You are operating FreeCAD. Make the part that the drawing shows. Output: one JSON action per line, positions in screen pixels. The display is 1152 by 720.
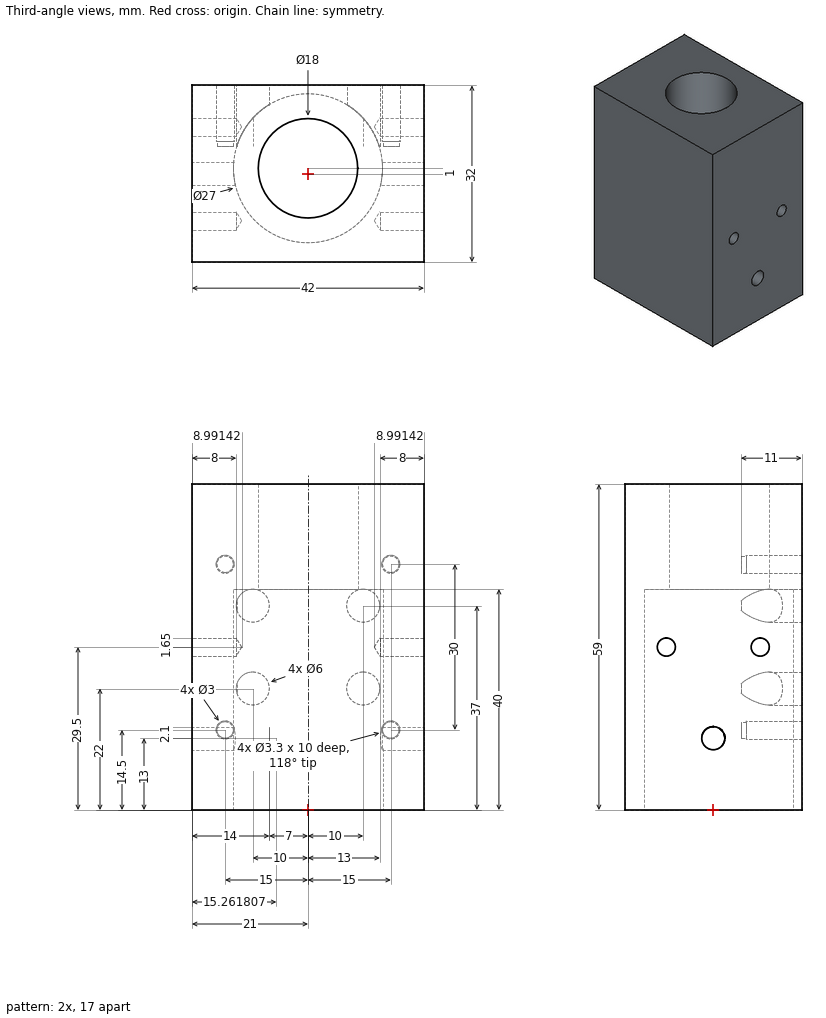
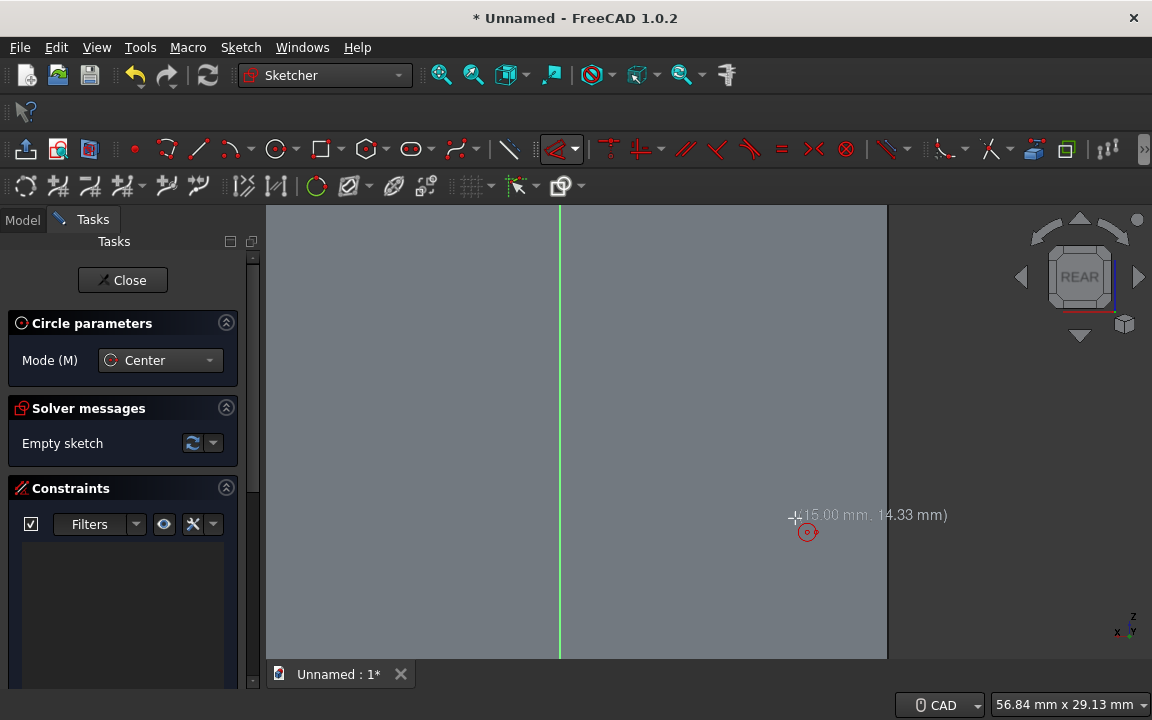
{"action": "left_click", "coordinate": [794, 517]}
{"action": "left_click", "coordinate": [811, 500]}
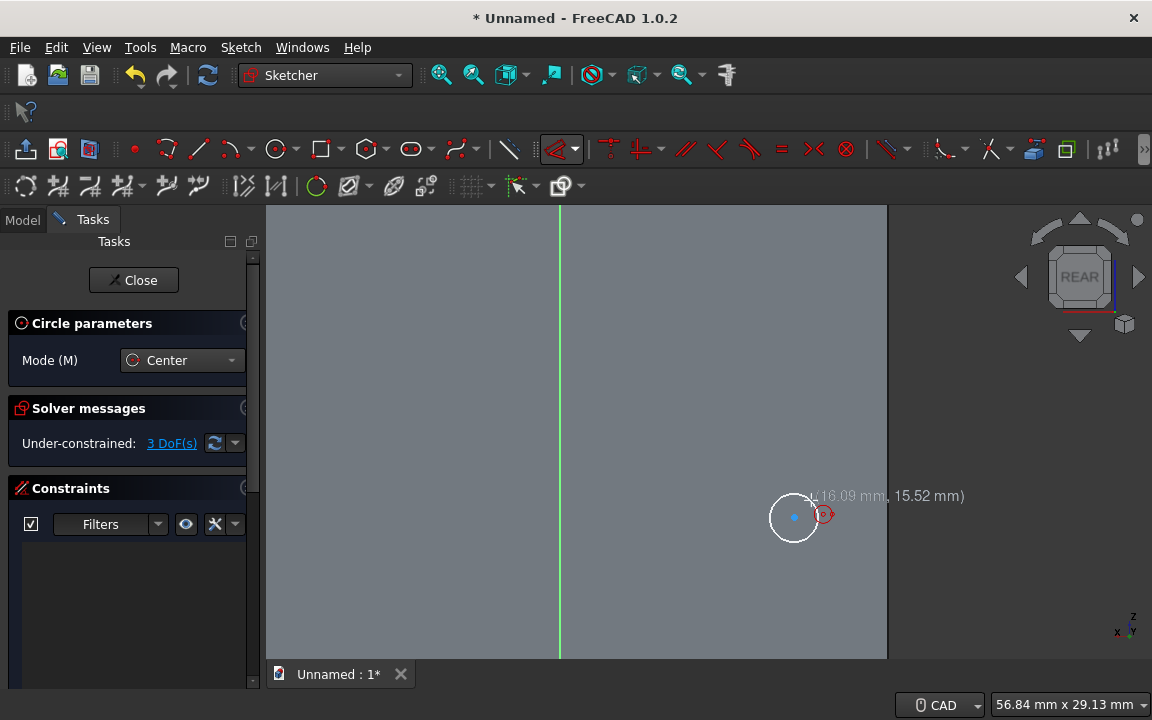
{"action": "left_click", "coordinate": [716, 400]}
{"action": "left_click", "coordinate": [749, 367]}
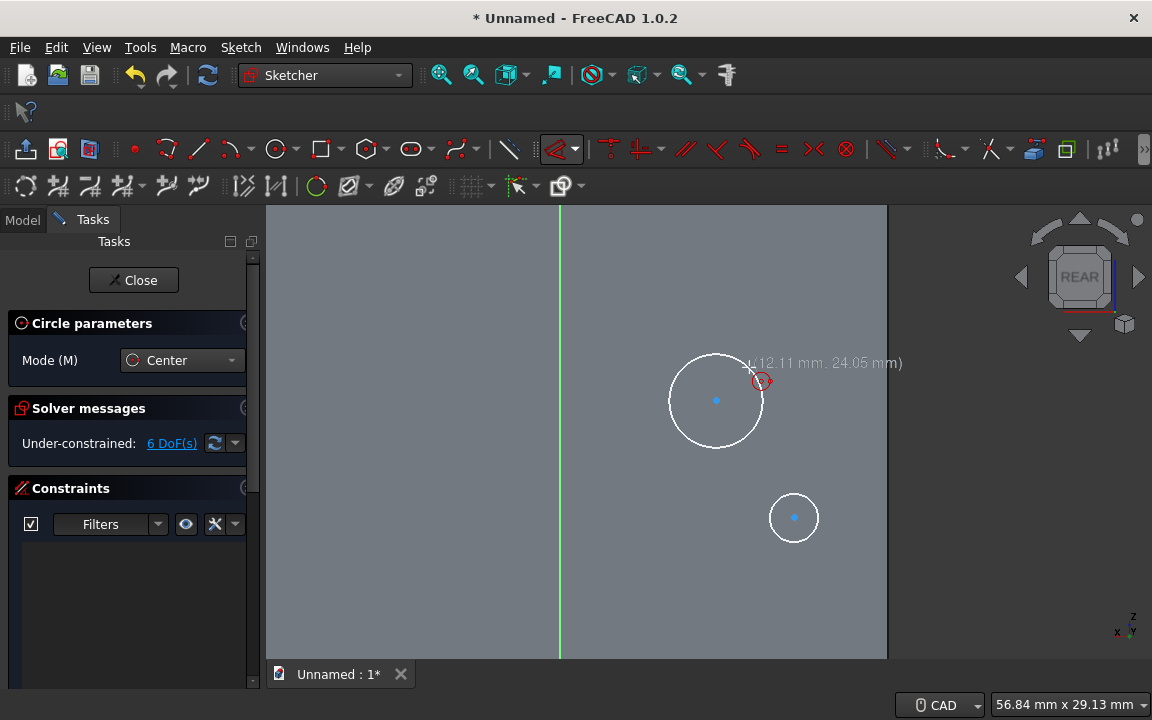
{"action": "left_click", "coordinate": [404, 400]}
{"action": "left_click", "coordinate": [437, 367]}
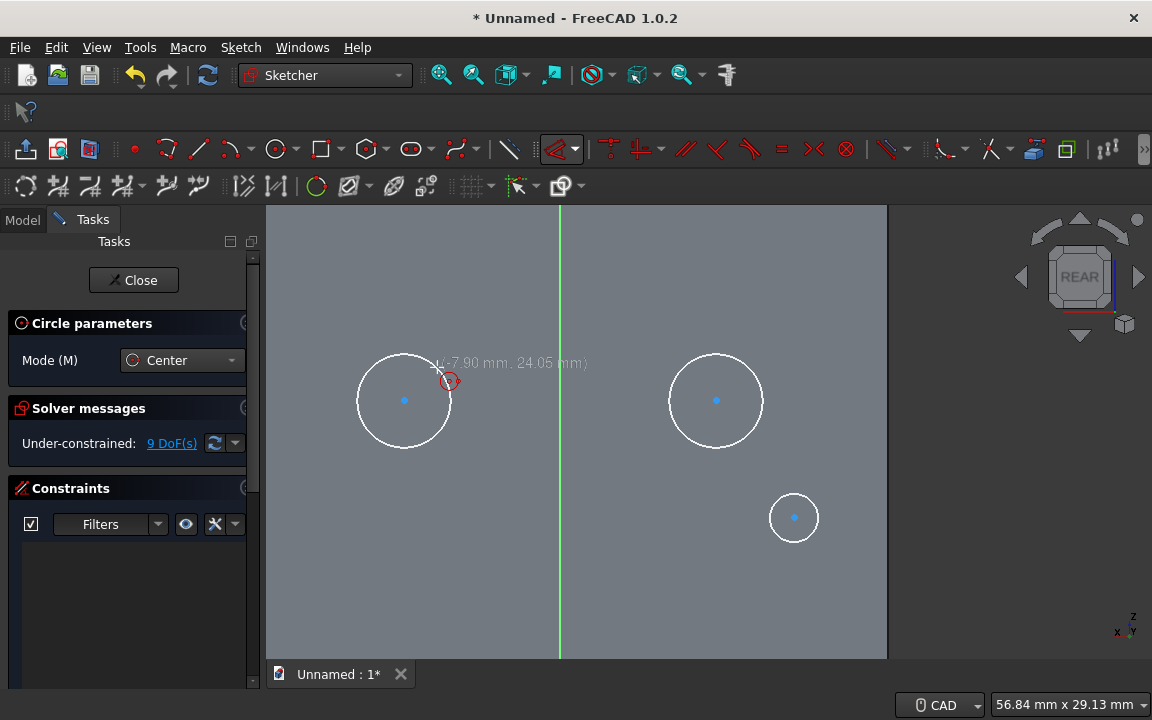
{"action": "left_click", "coordinate": [326, 517]}
{"action": "left_click", "coordinate": [343, 500]}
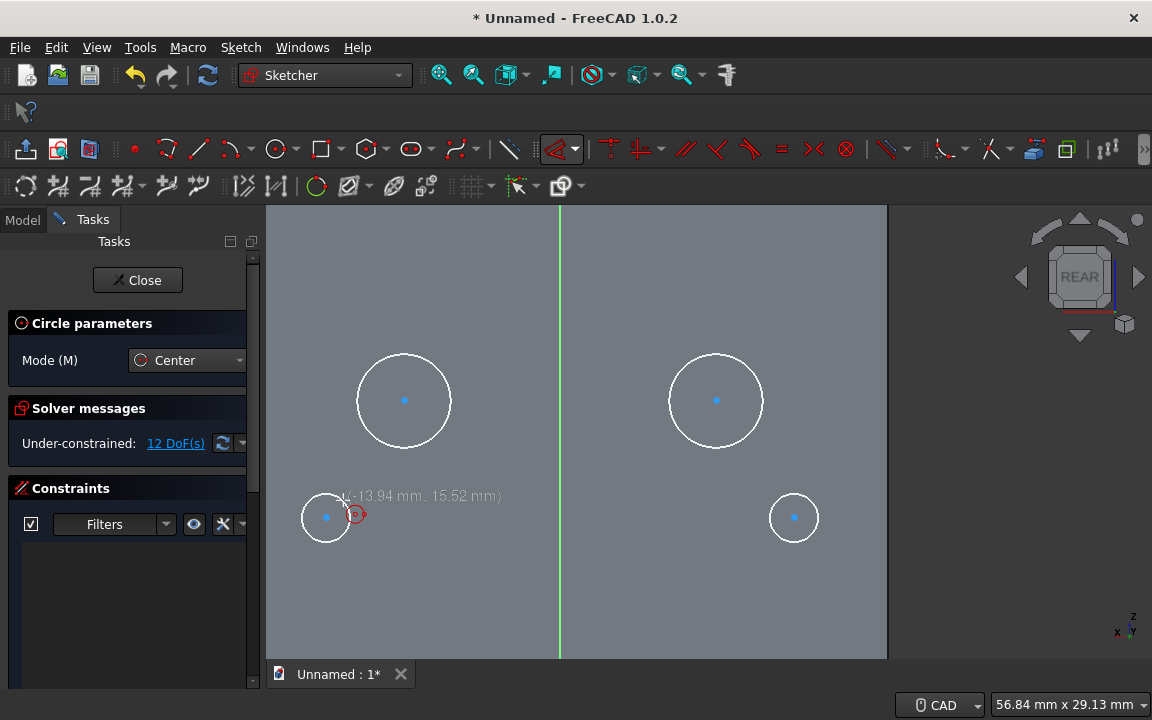
{"action": "scroll", "coordinate": [687, 460], "scroll_direction": "down", "scroll_amount": 5}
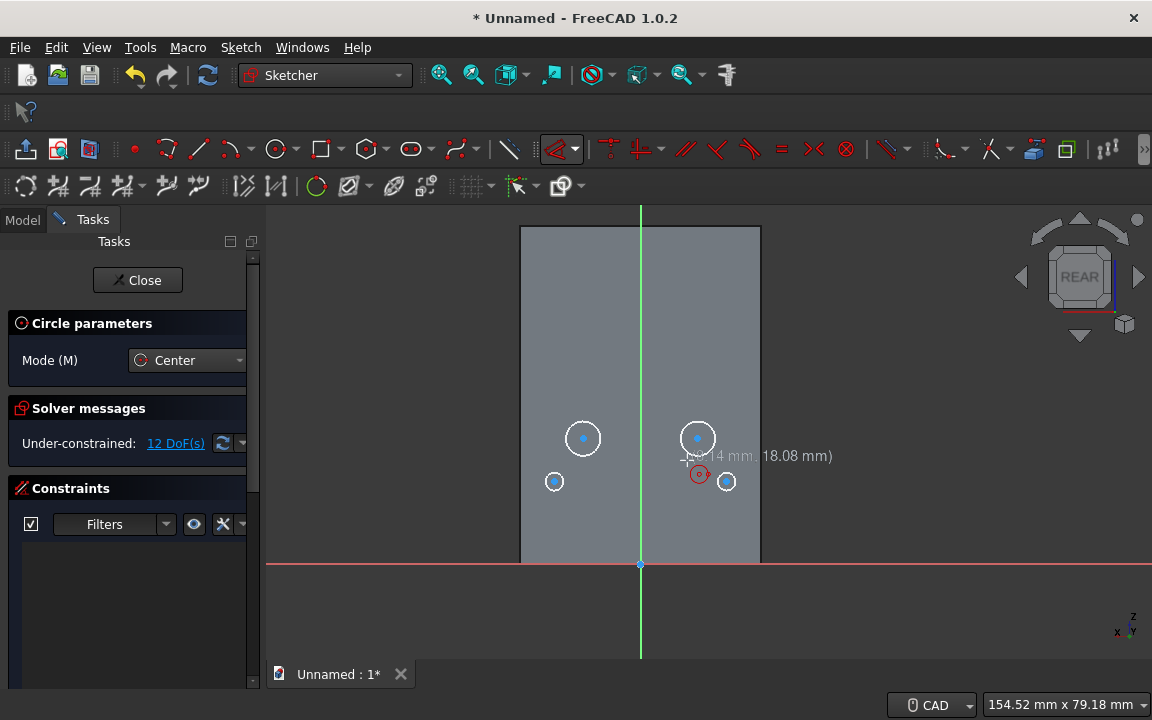
{"action": "scroll", "coordinate": [555, 309], "scroll_direction": "up", "scroll_amount": 5}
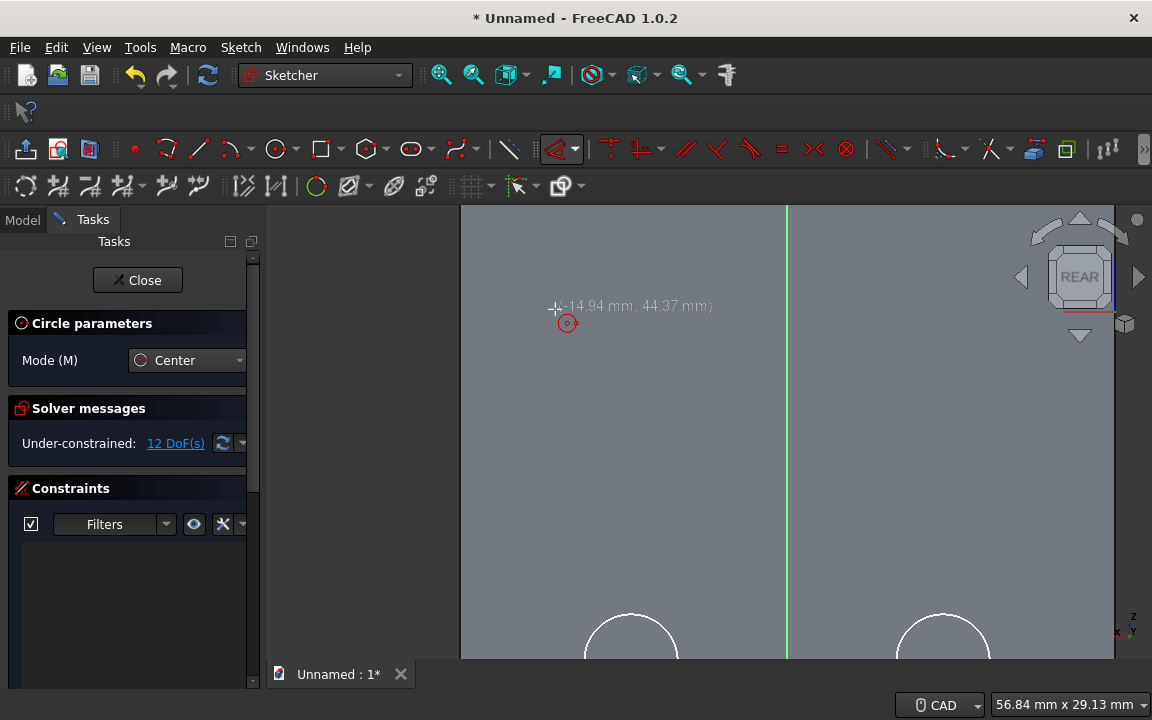
{"action": "left_click", "coordinate": [553, 309]}
{"action": "left_click", "coordinate": [570, 293]}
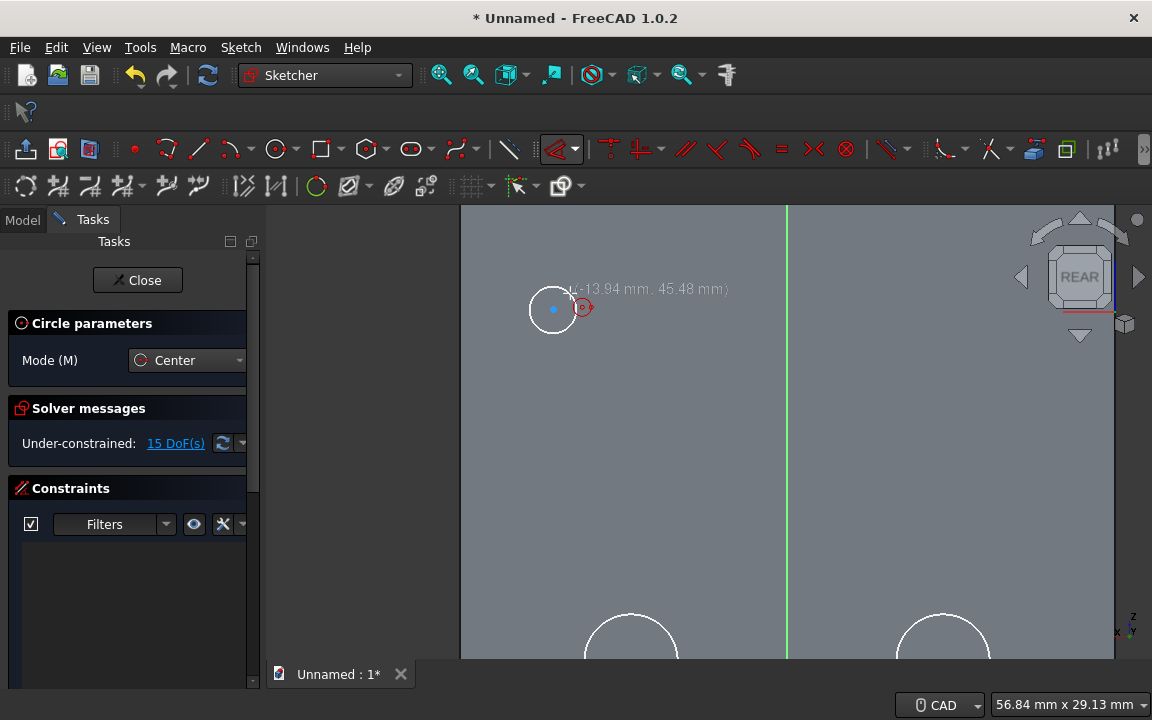
{"action": "left_click", "coordinate": [631, 426]}
{"action": "left_click", "coordinate": [664, 393]}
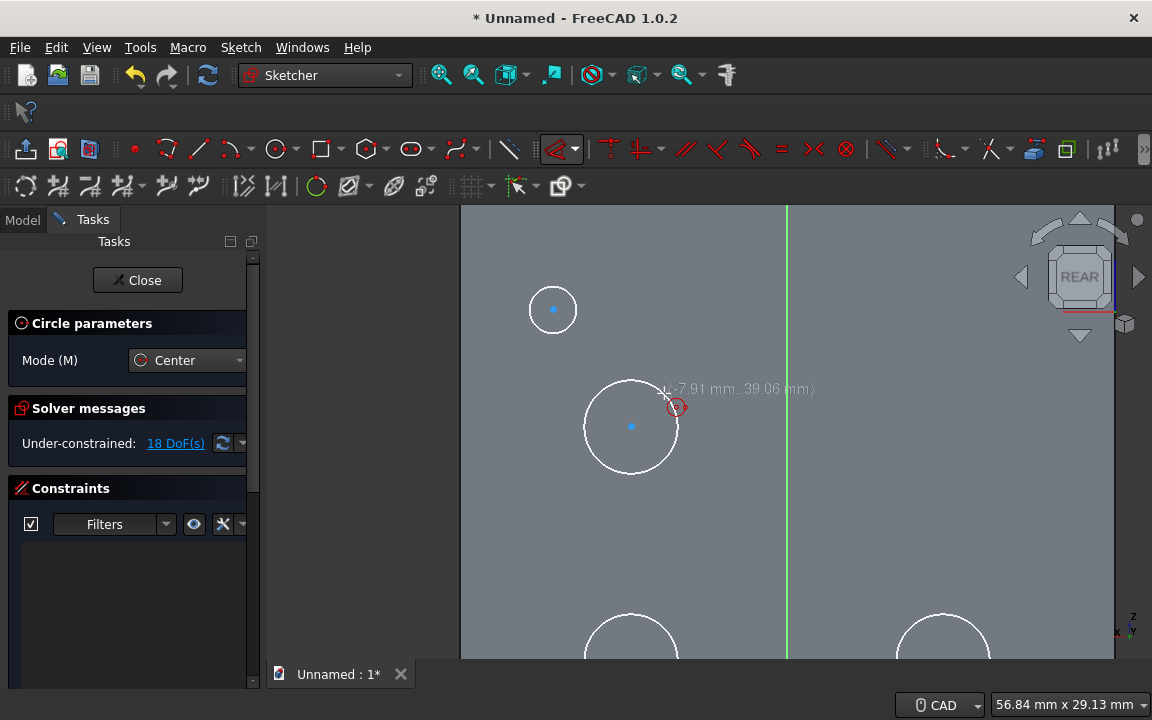
{"action": "left_click", "coordinate": [943, 426]}
{"action": "left_click", "coordinate": [976, 393]}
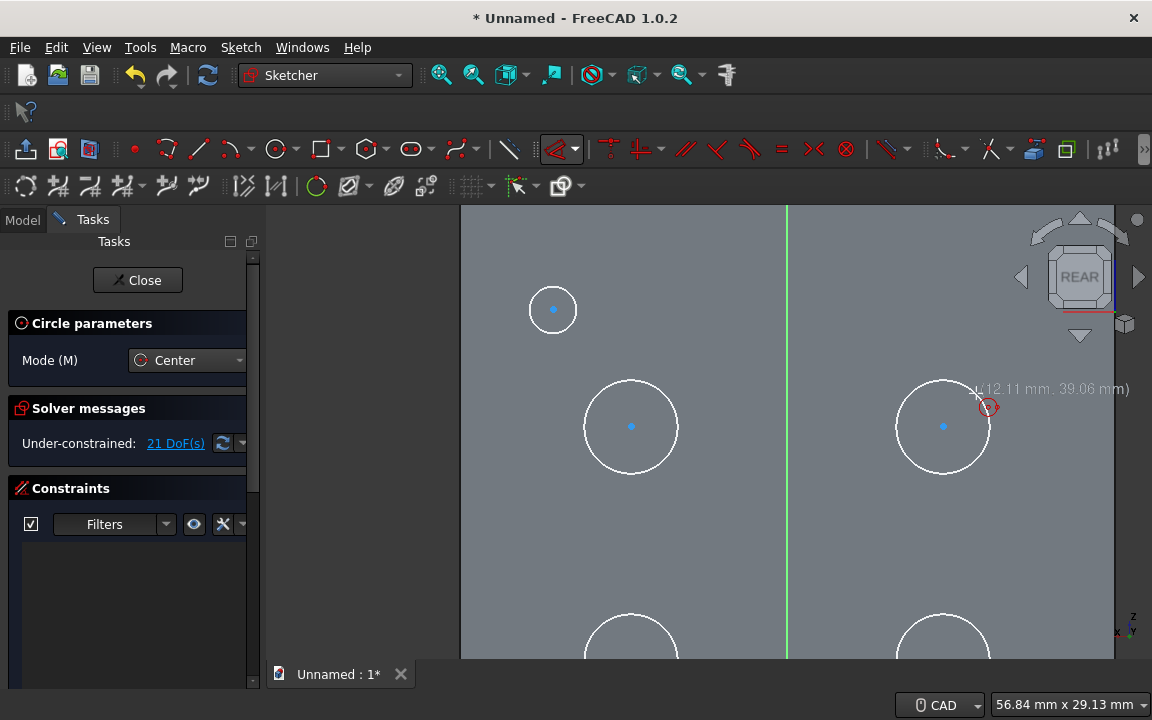
{"action": "scroll", "coordinate": [555, 308], "scroll_direction": "down", "scroll_amount": 5}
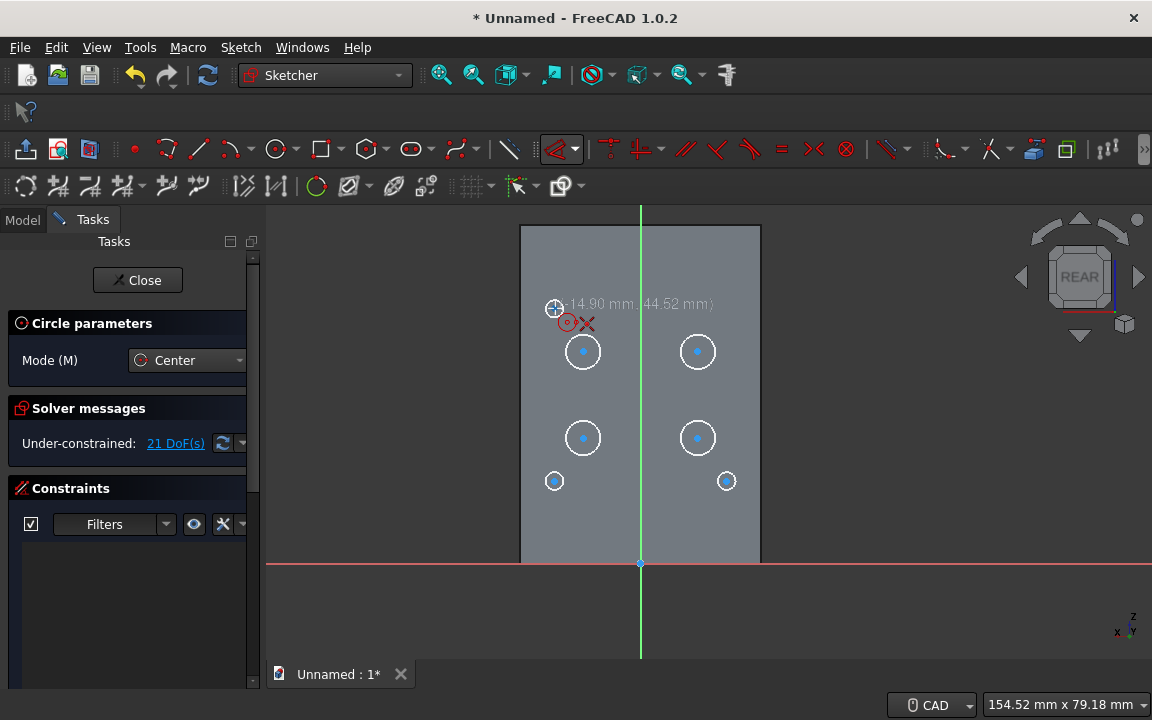
{"action": "scroll", "coordinate": [727, 309], "scroll_direction": "up", "scroll_amount": 5}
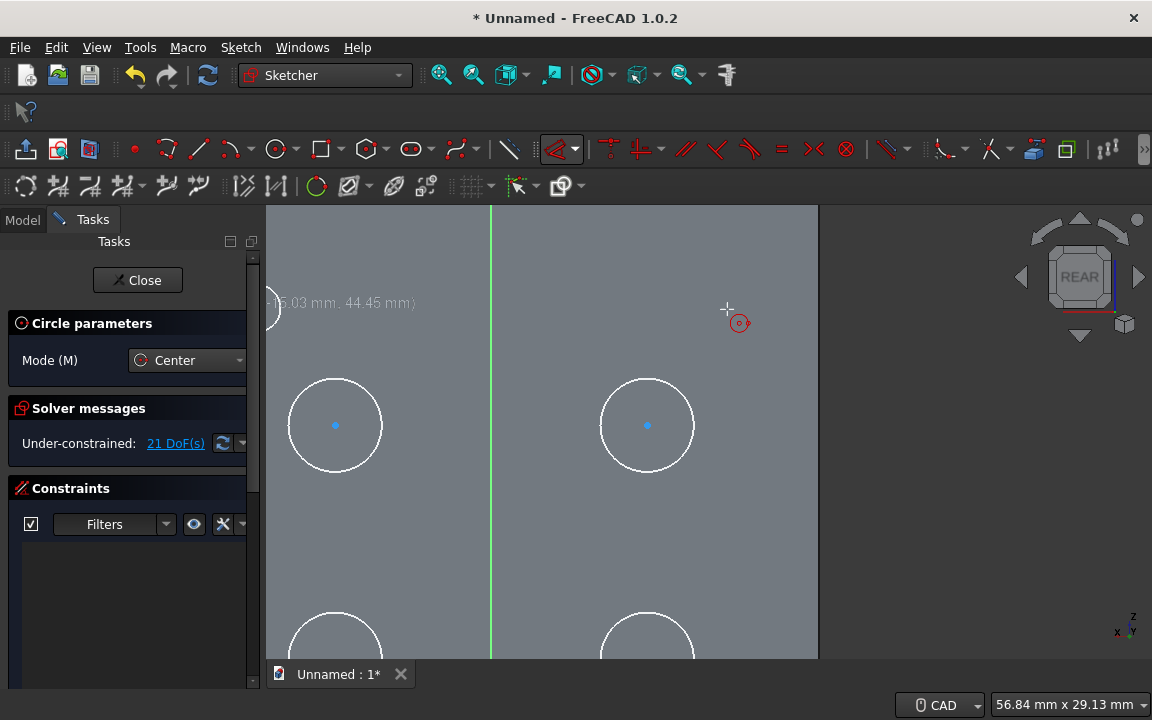
{"action": "left_click", "coordinate": [725, 308]}
{"action": "left_click", "coordinate": [742, 291]}
{"action": "key", "text": "Escape"}